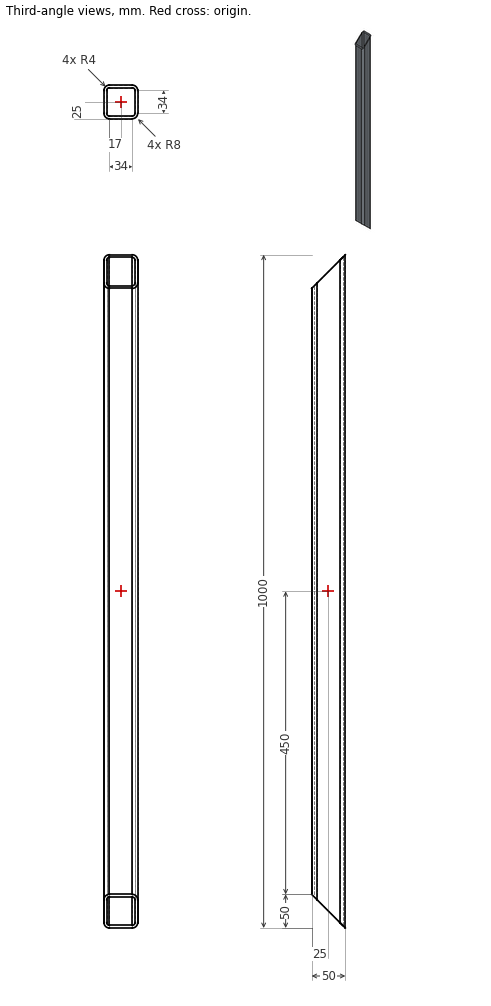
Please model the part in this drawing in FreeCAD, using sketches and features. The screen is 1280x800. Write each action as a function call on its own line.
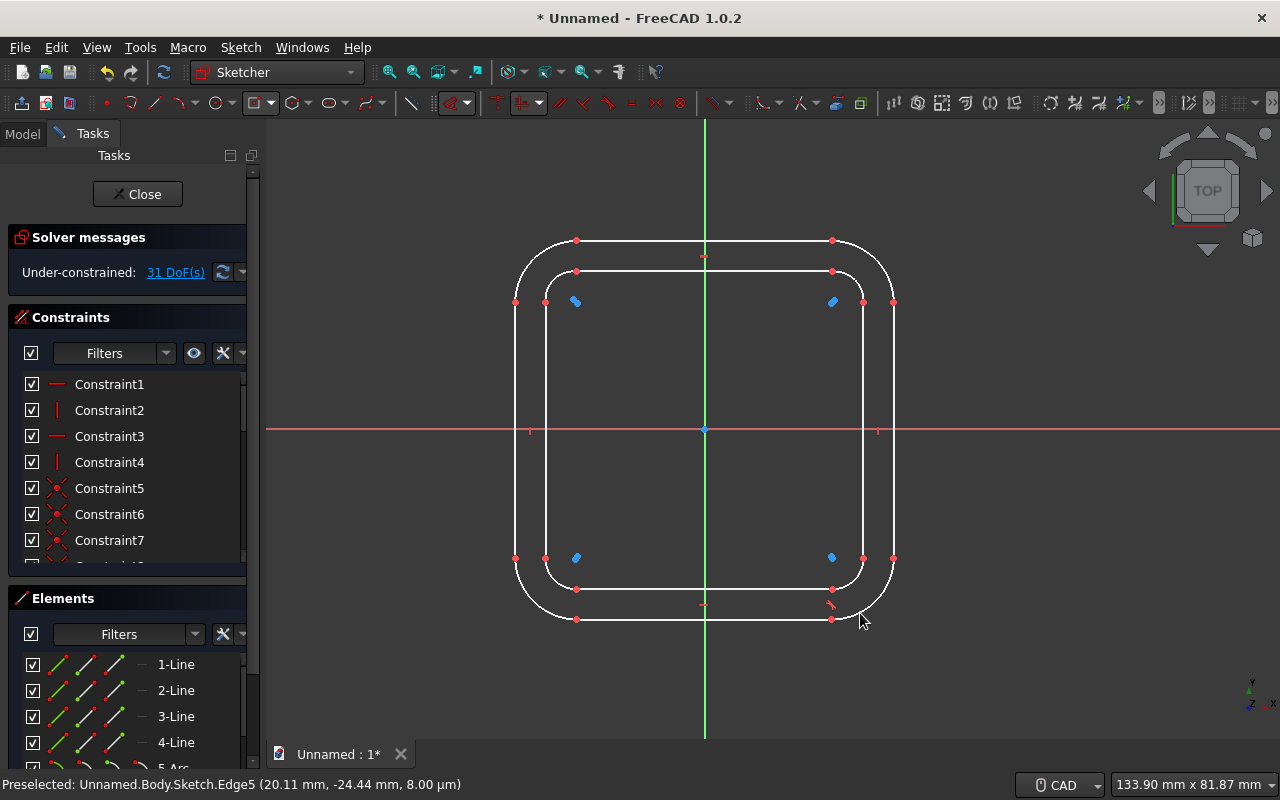
click(653, 620)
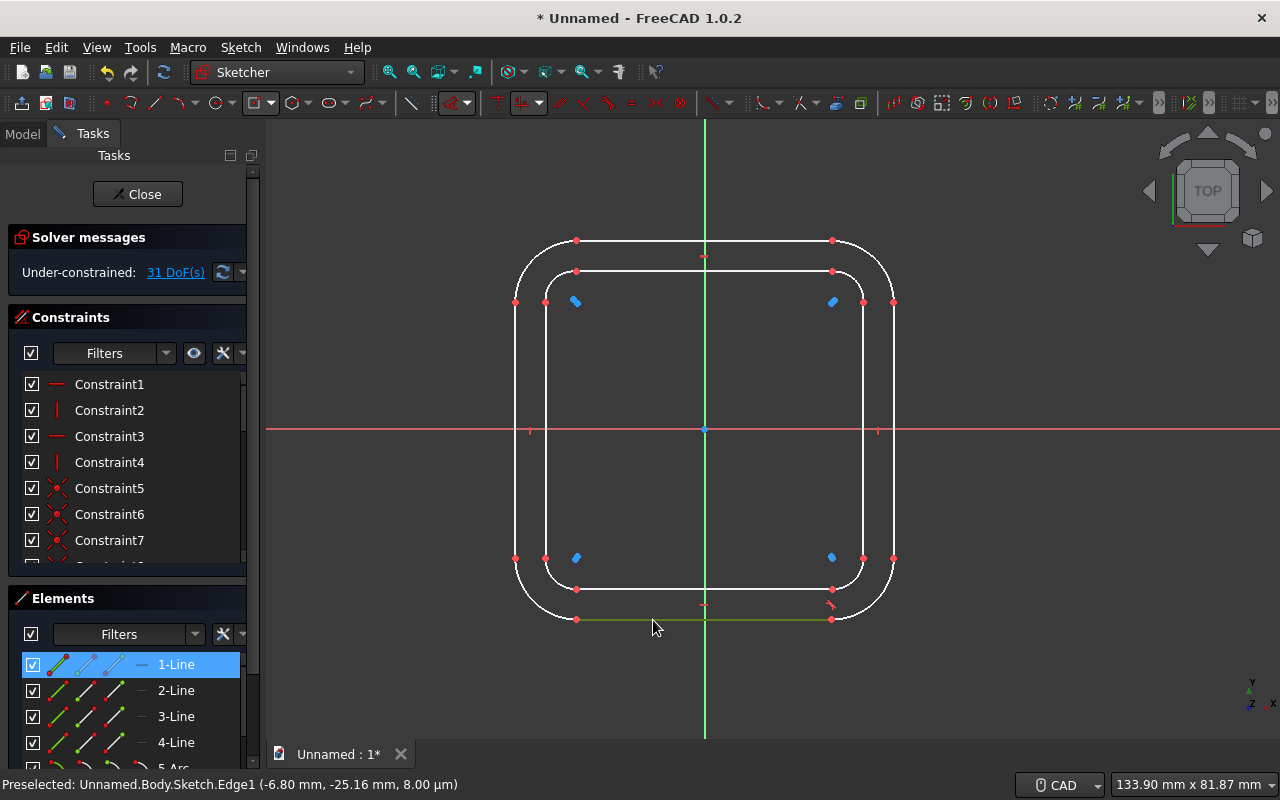
click(522, 586)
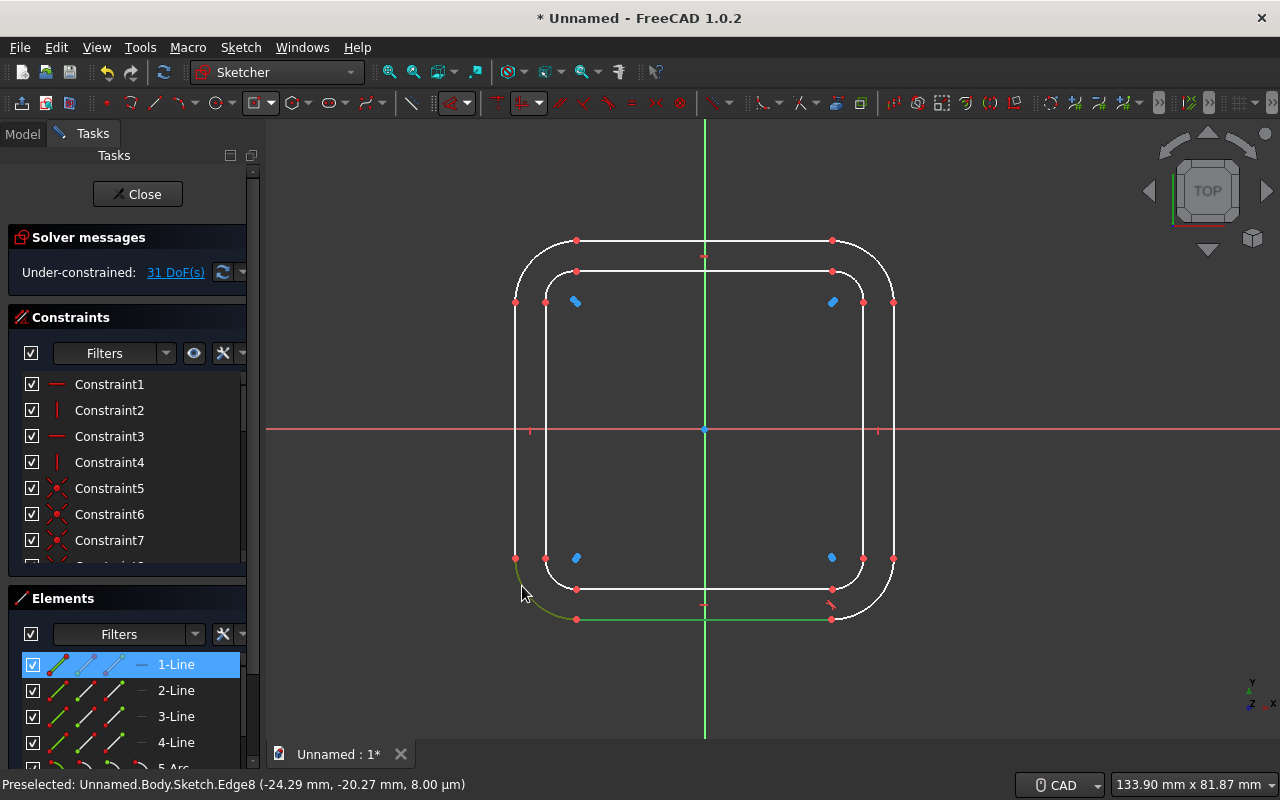
key(t)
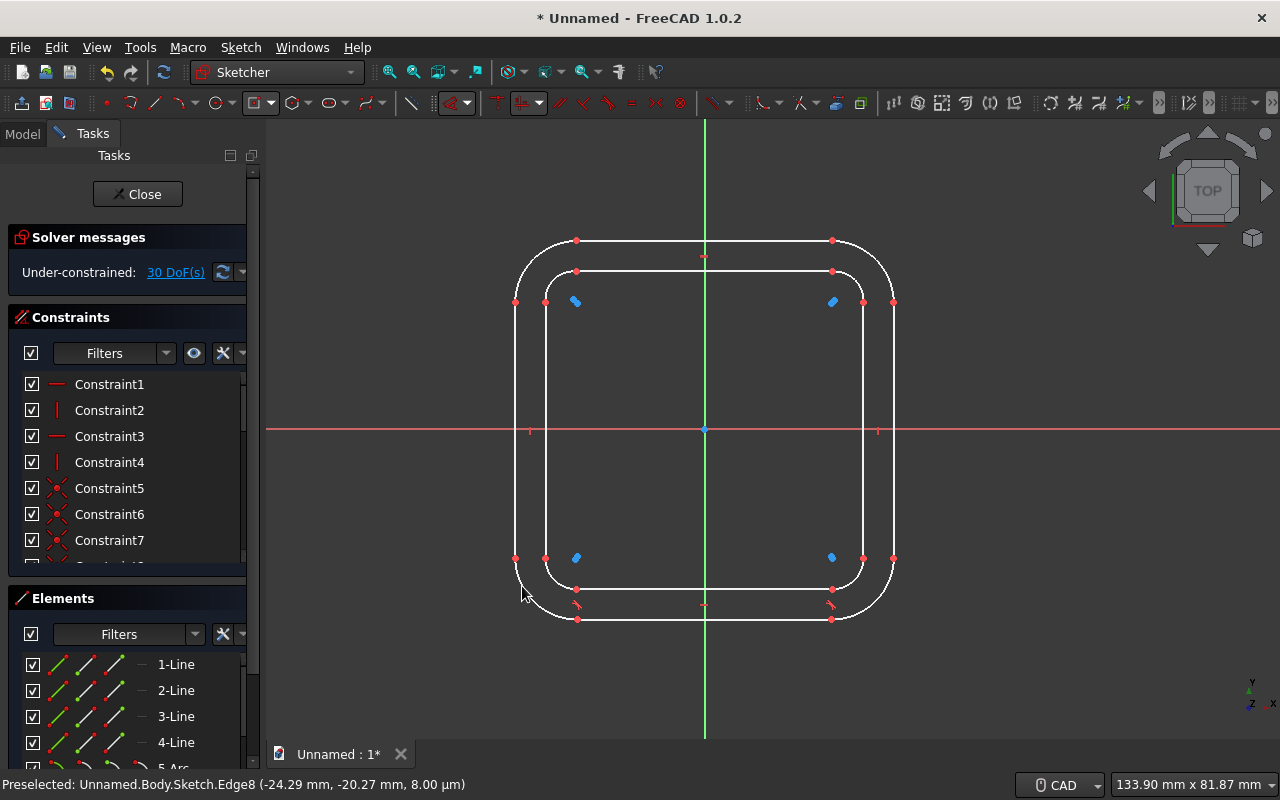
click(894, 482)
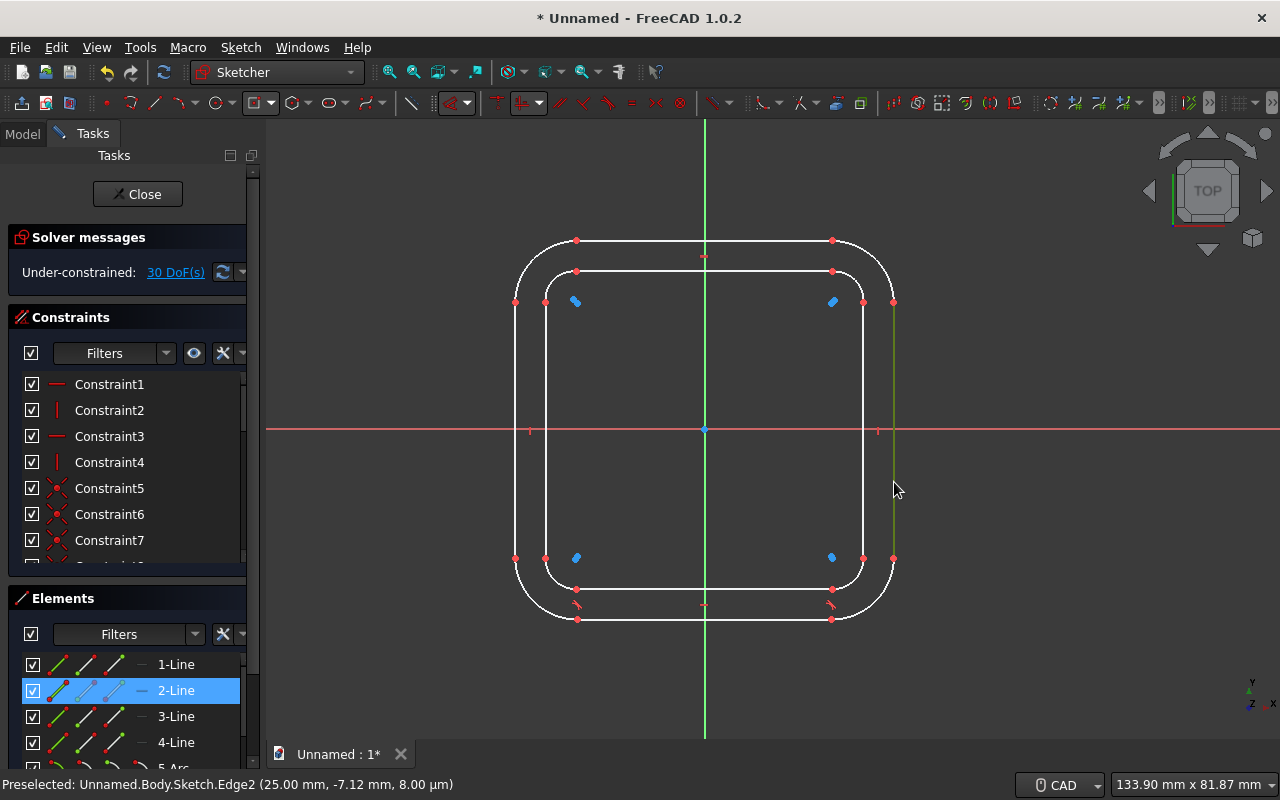
click(859, 613)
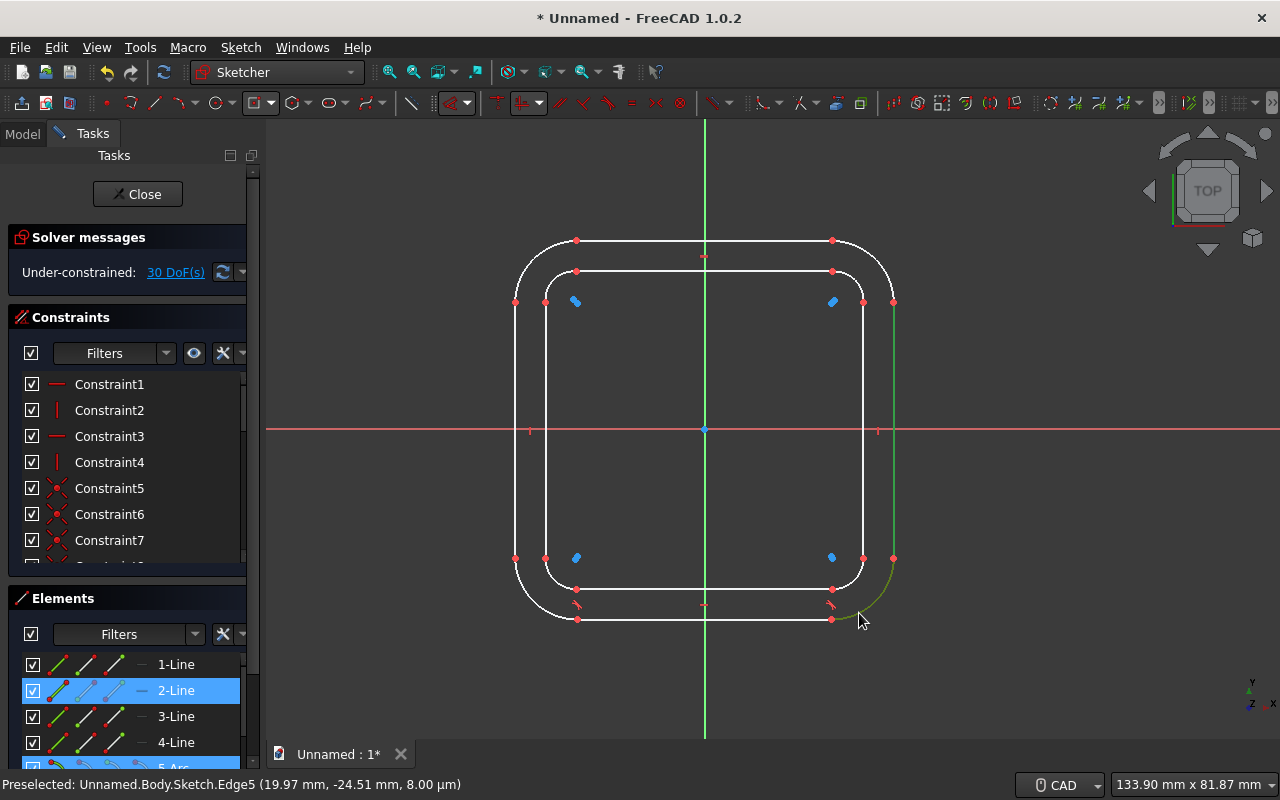
click(608, 104)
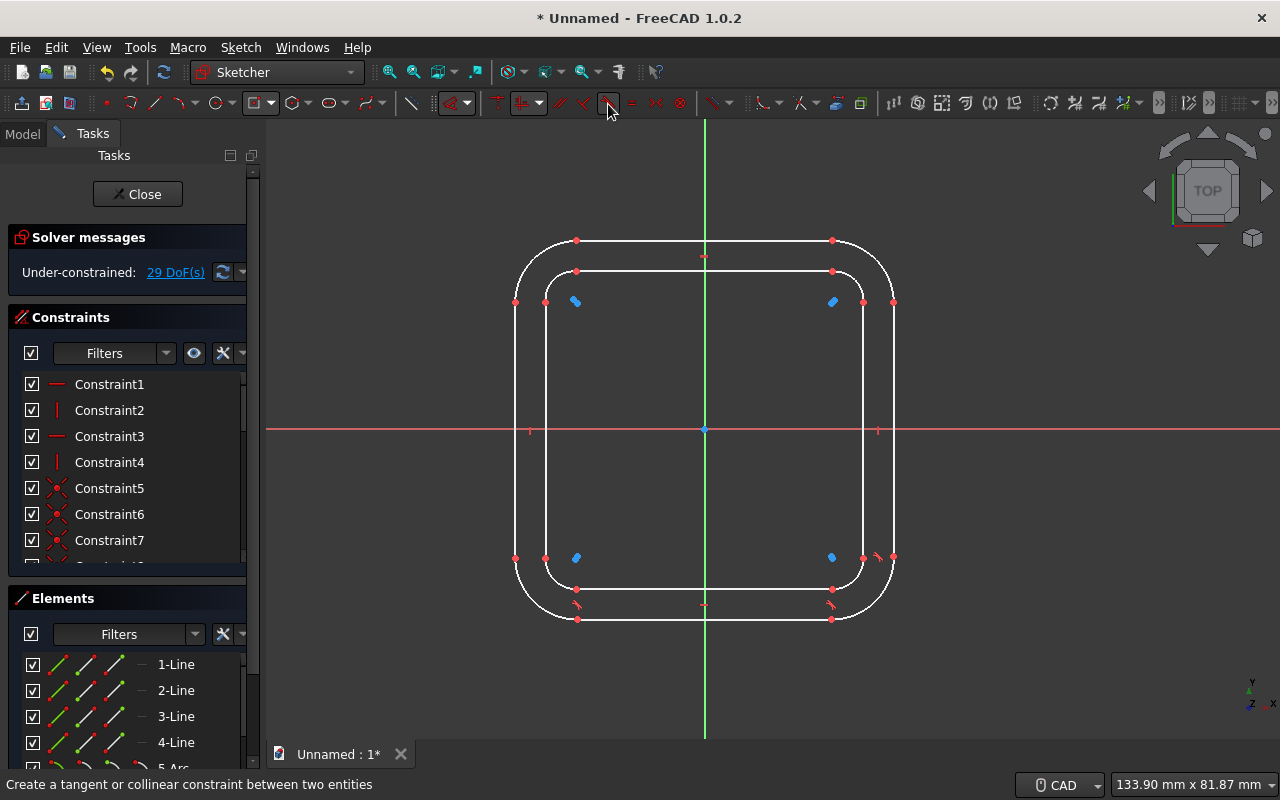
click(894, 481)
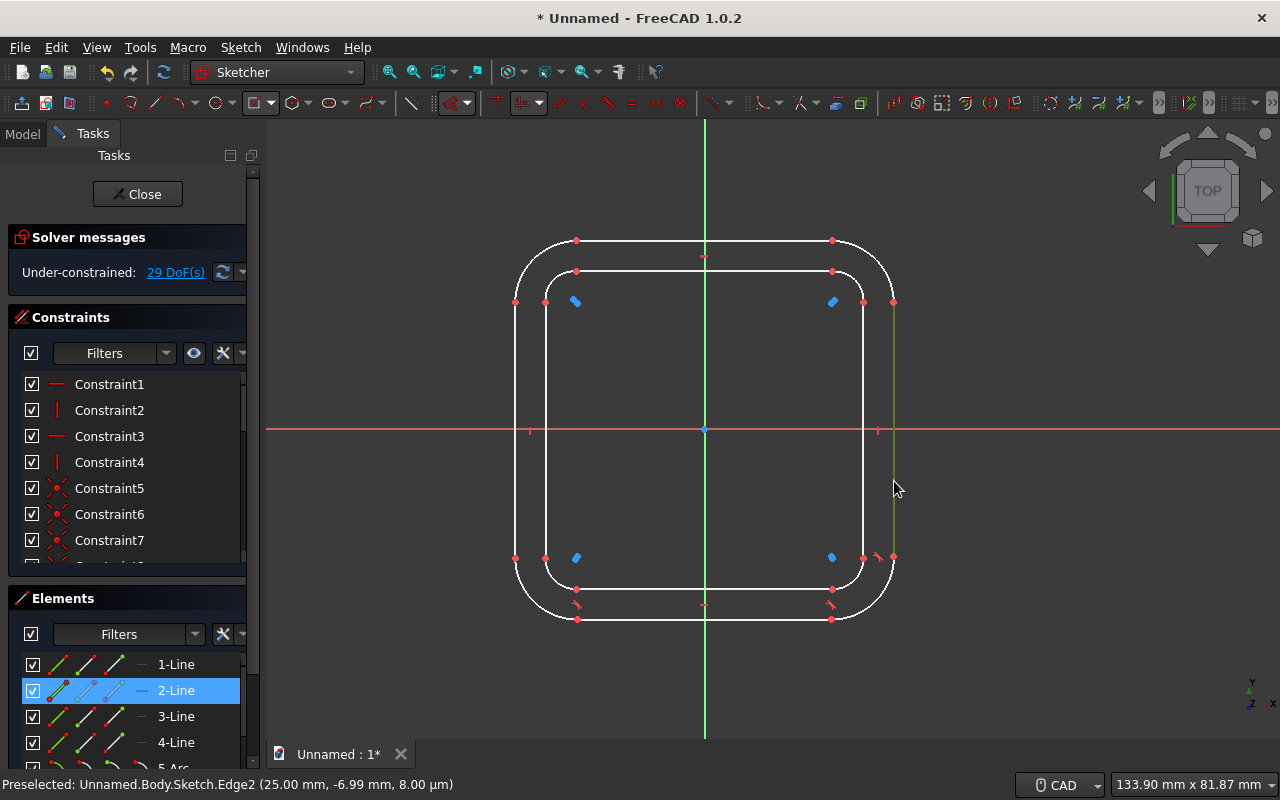
click(887, 275)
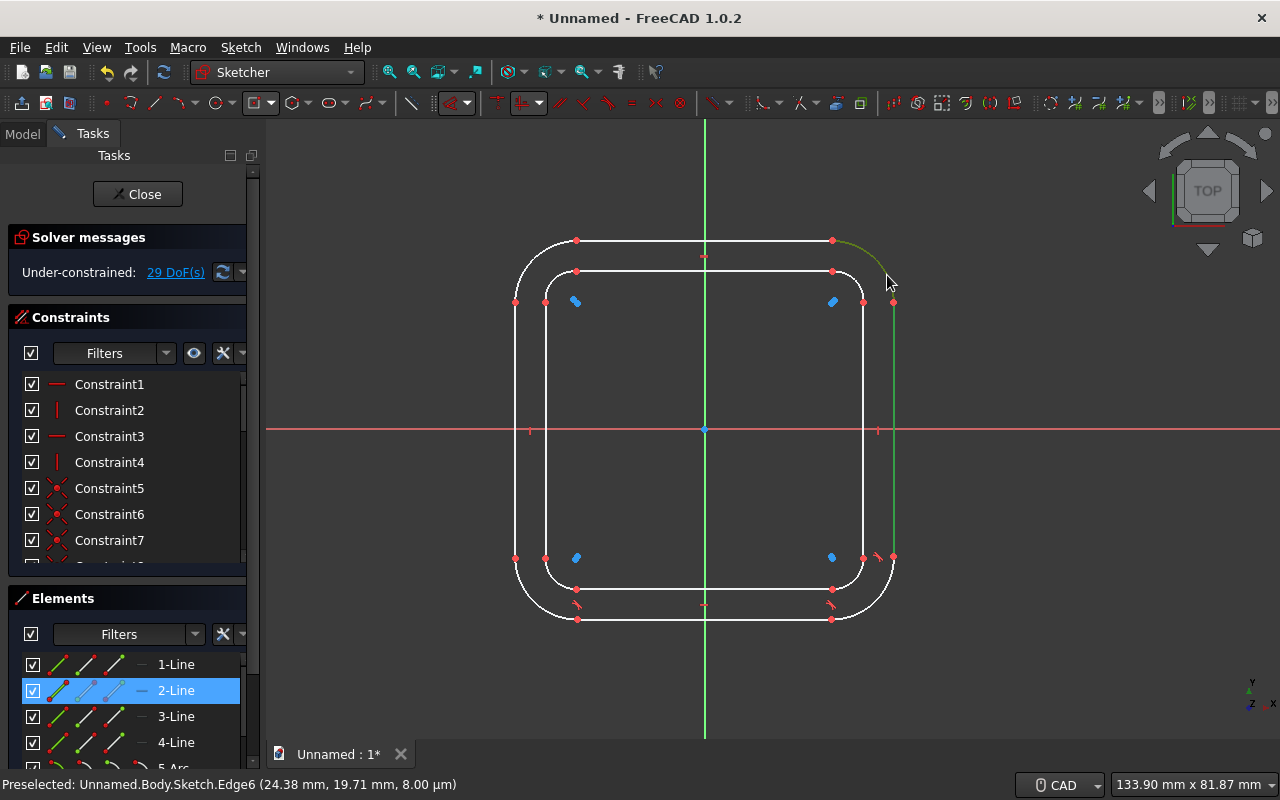
key(t)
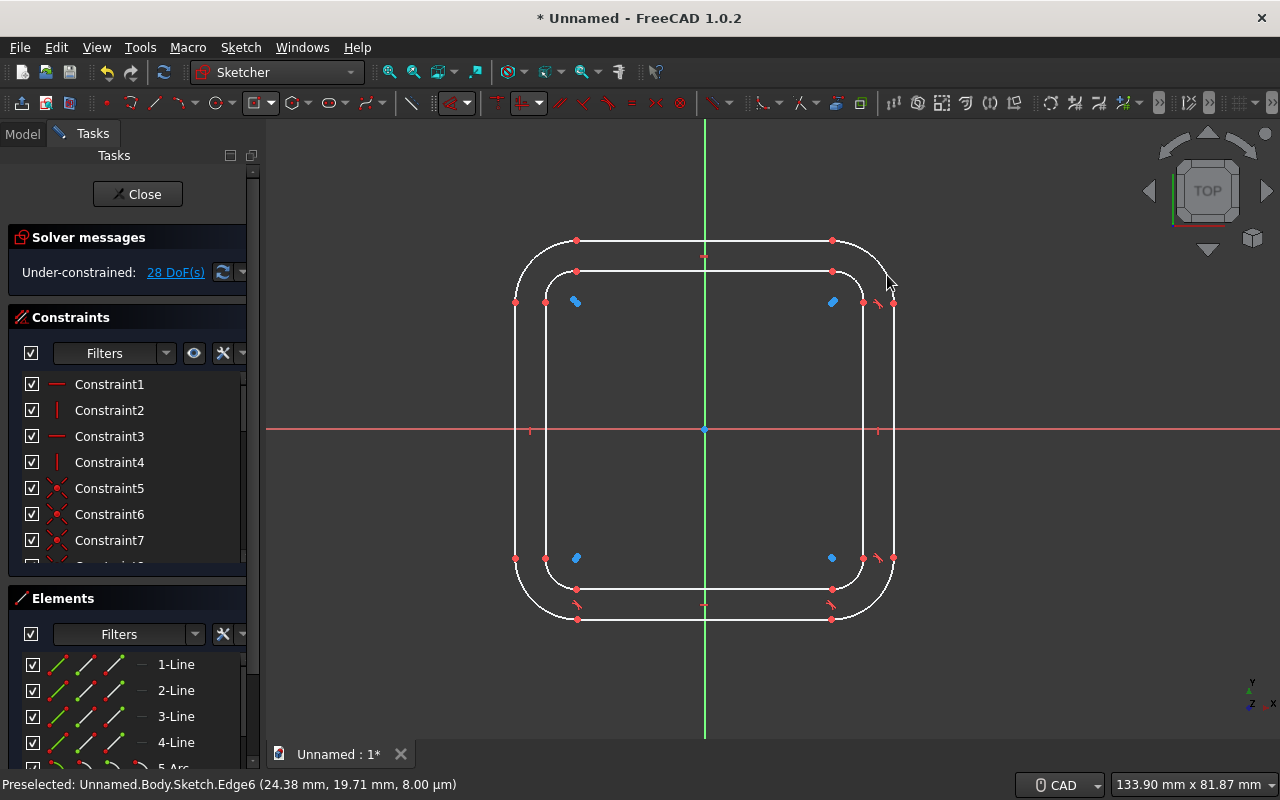
click(756, 241)